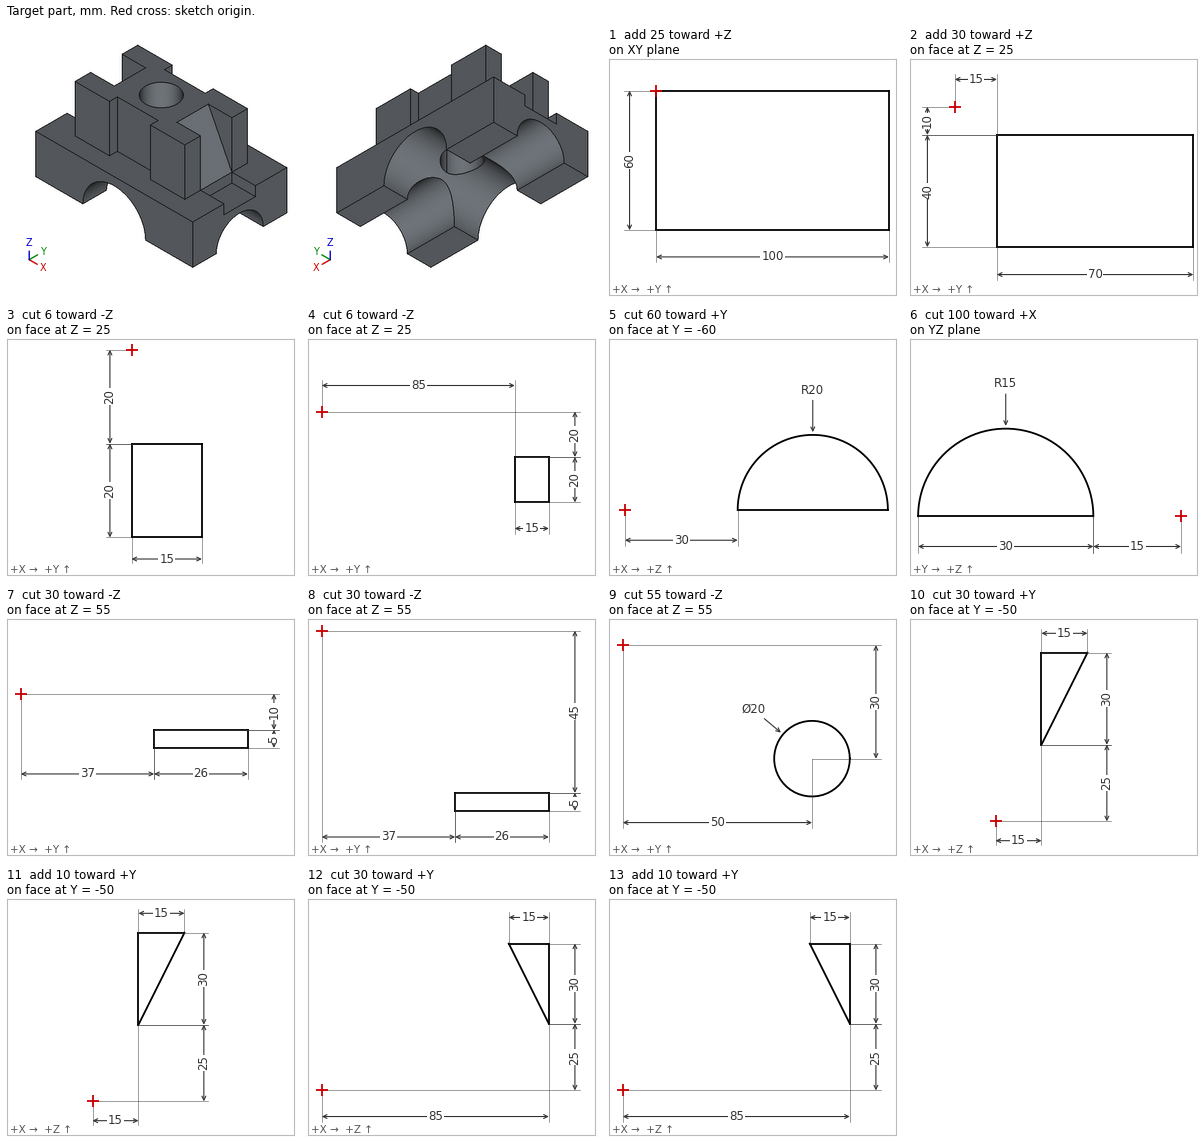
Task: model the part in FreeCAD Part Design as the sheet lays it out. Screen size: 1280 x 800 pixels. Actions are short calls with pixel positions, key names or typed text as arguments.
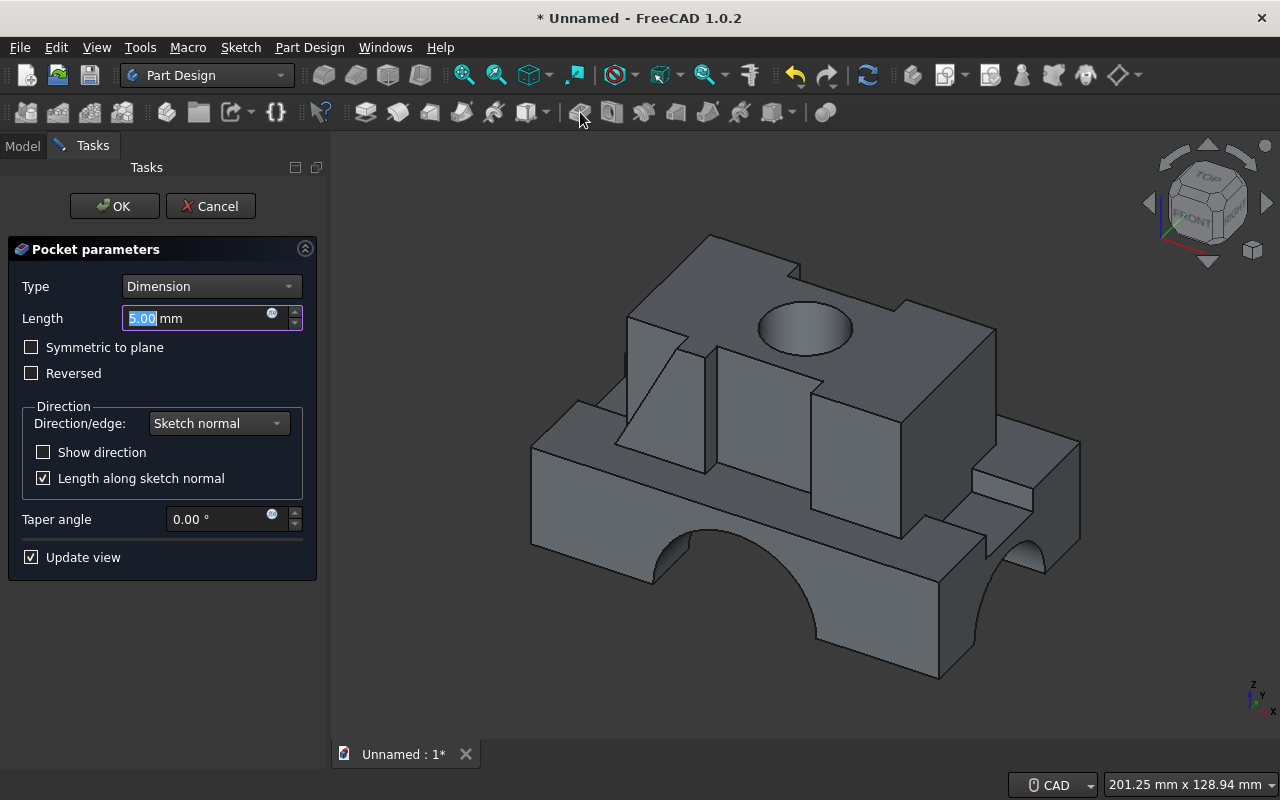
text(30)
key(Tab)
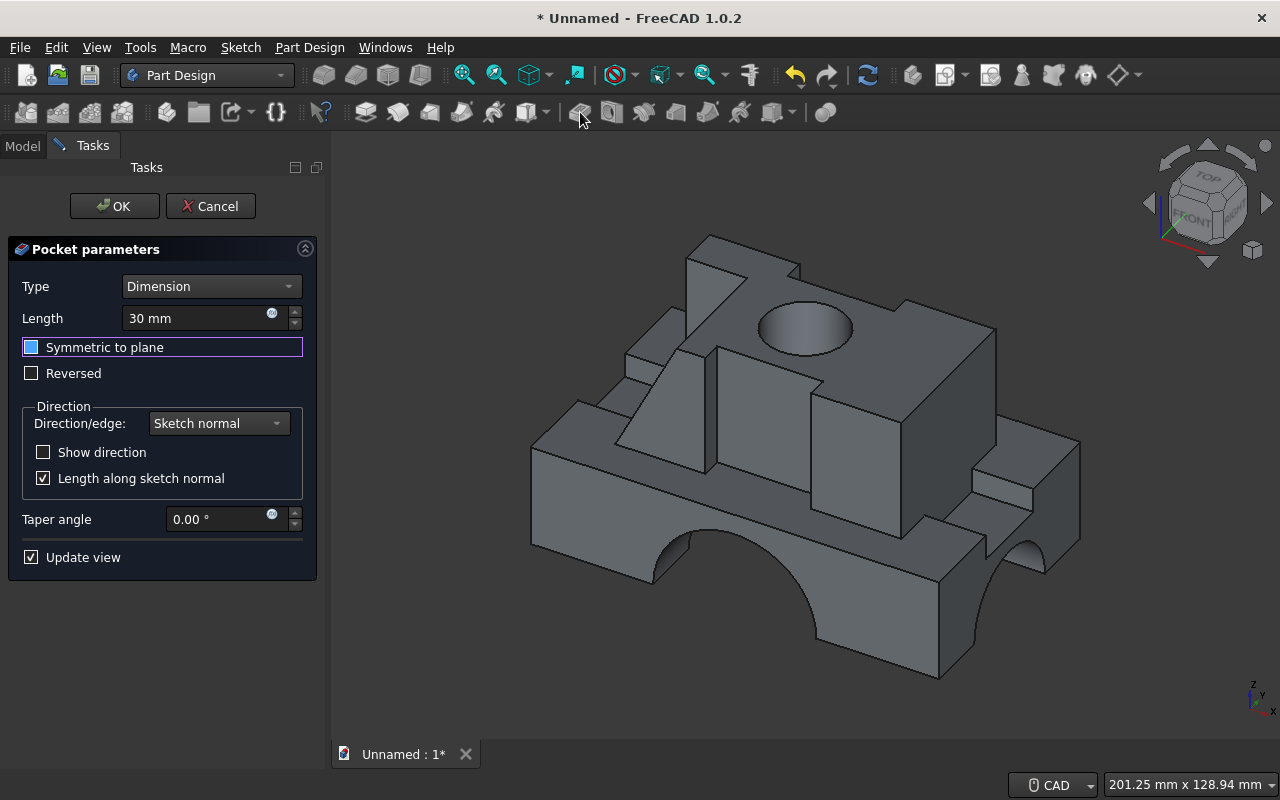
click(115, 206)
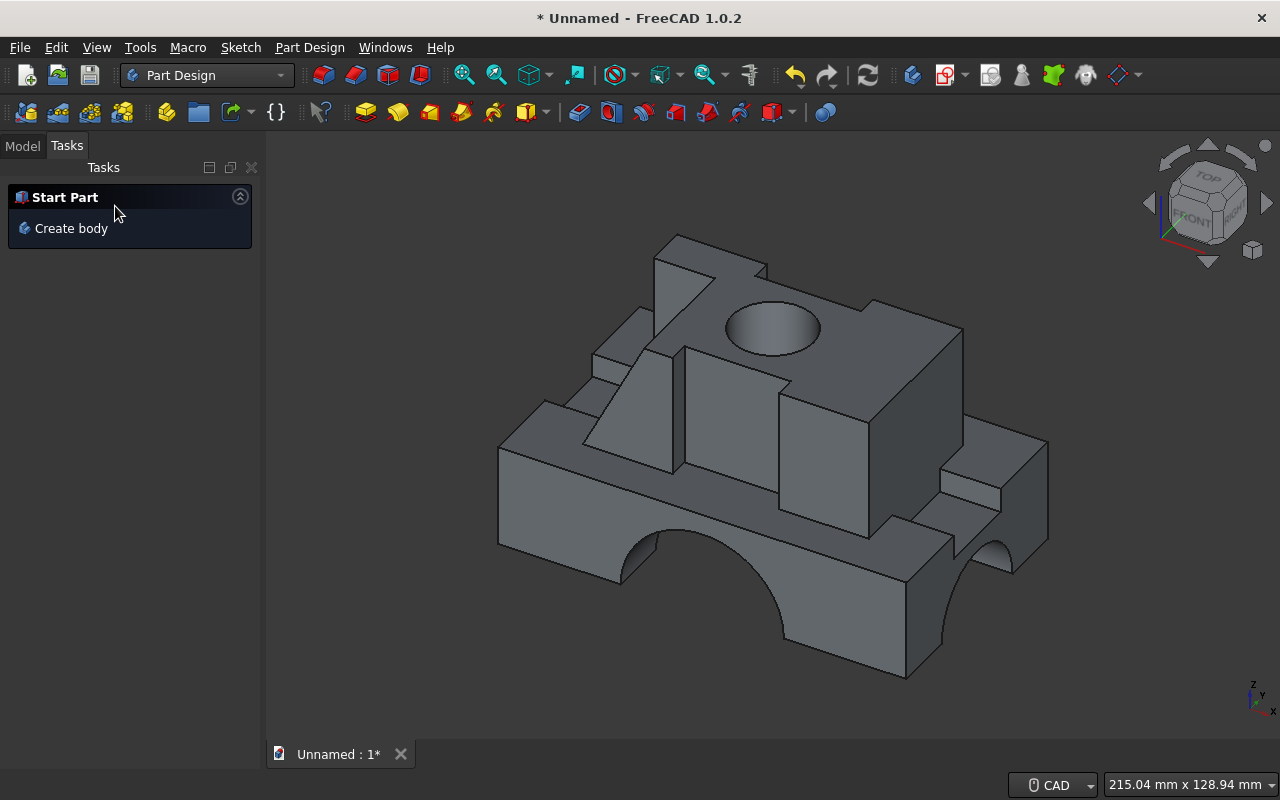
click(824, 465)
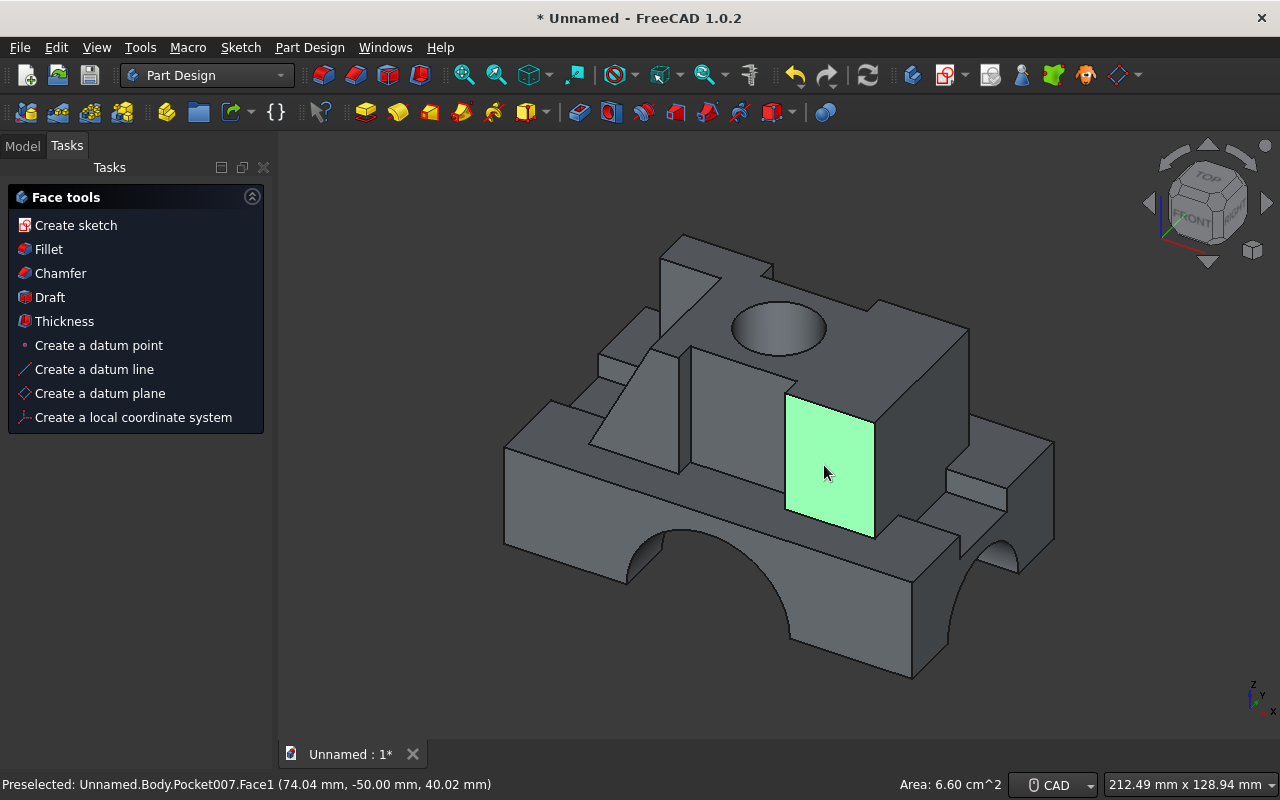
click(946, 76)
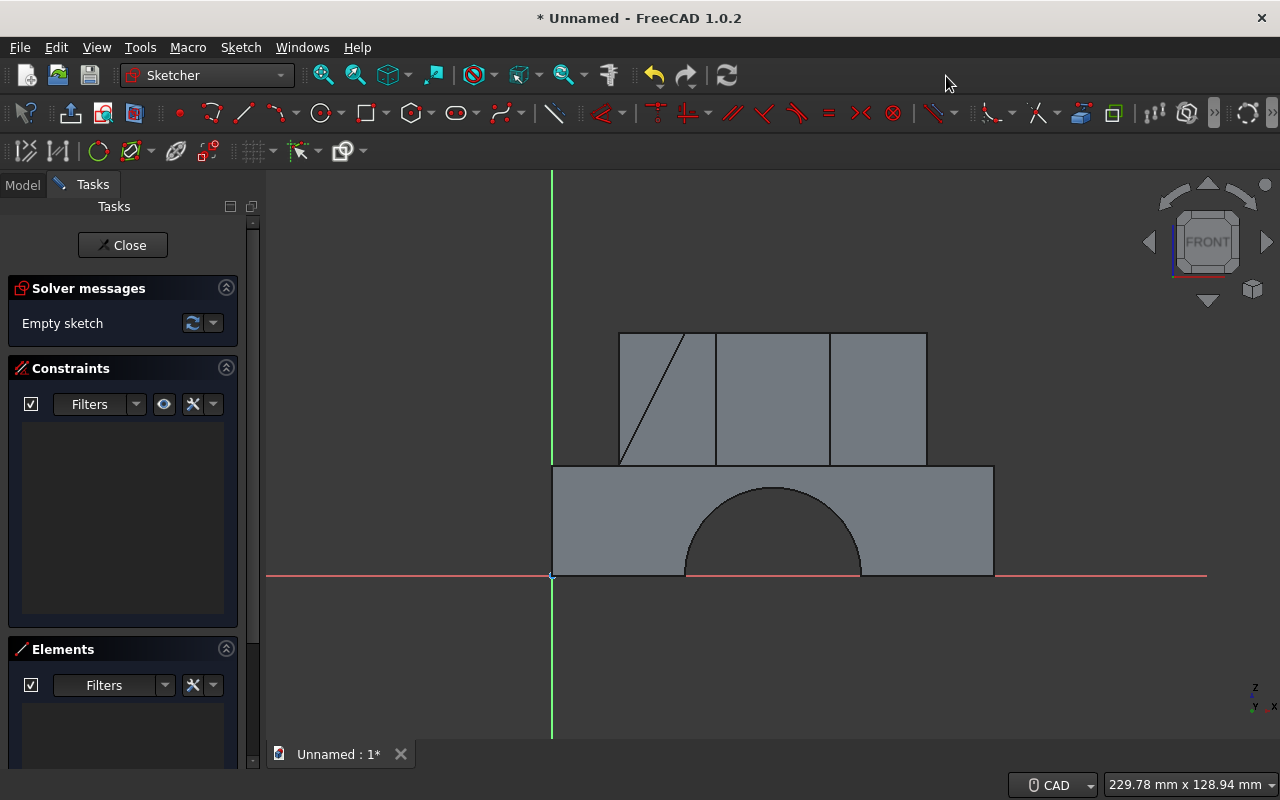
key(q)
key(s)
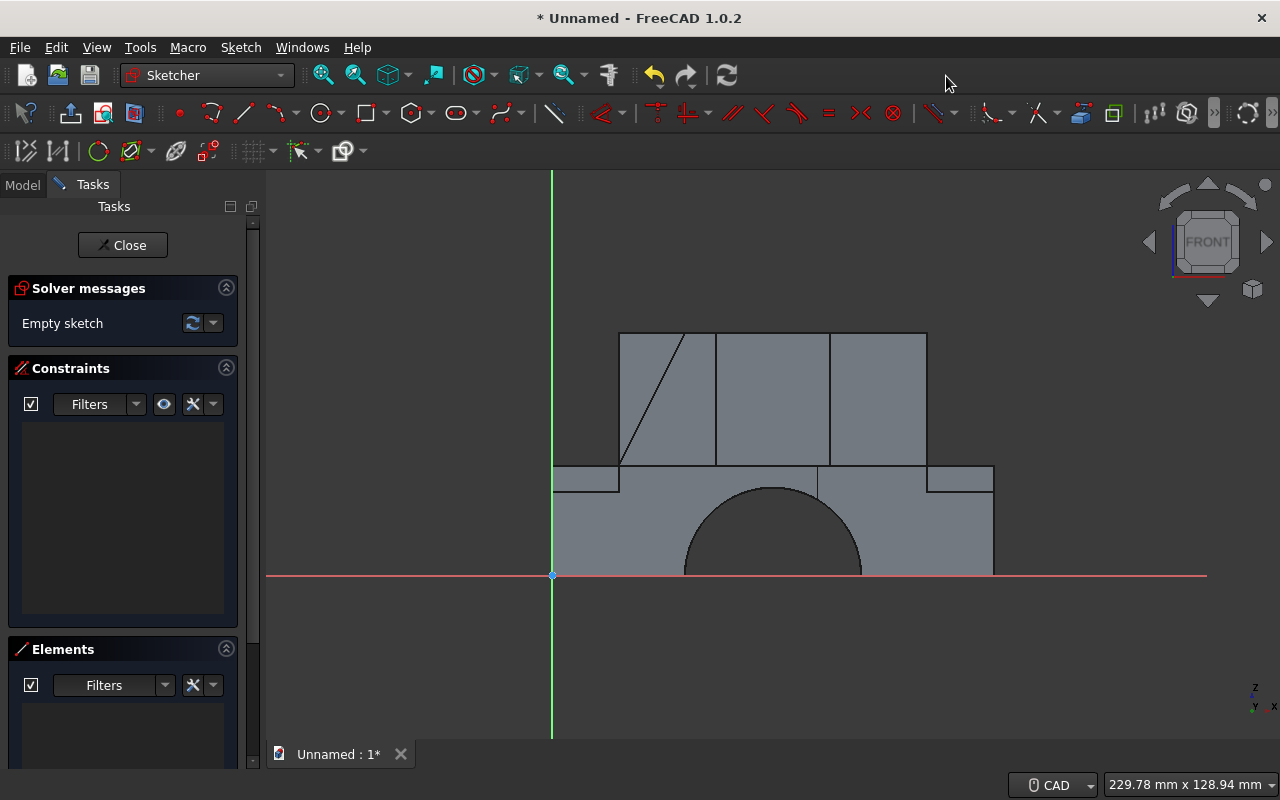
scroll(444, 454, up, 2)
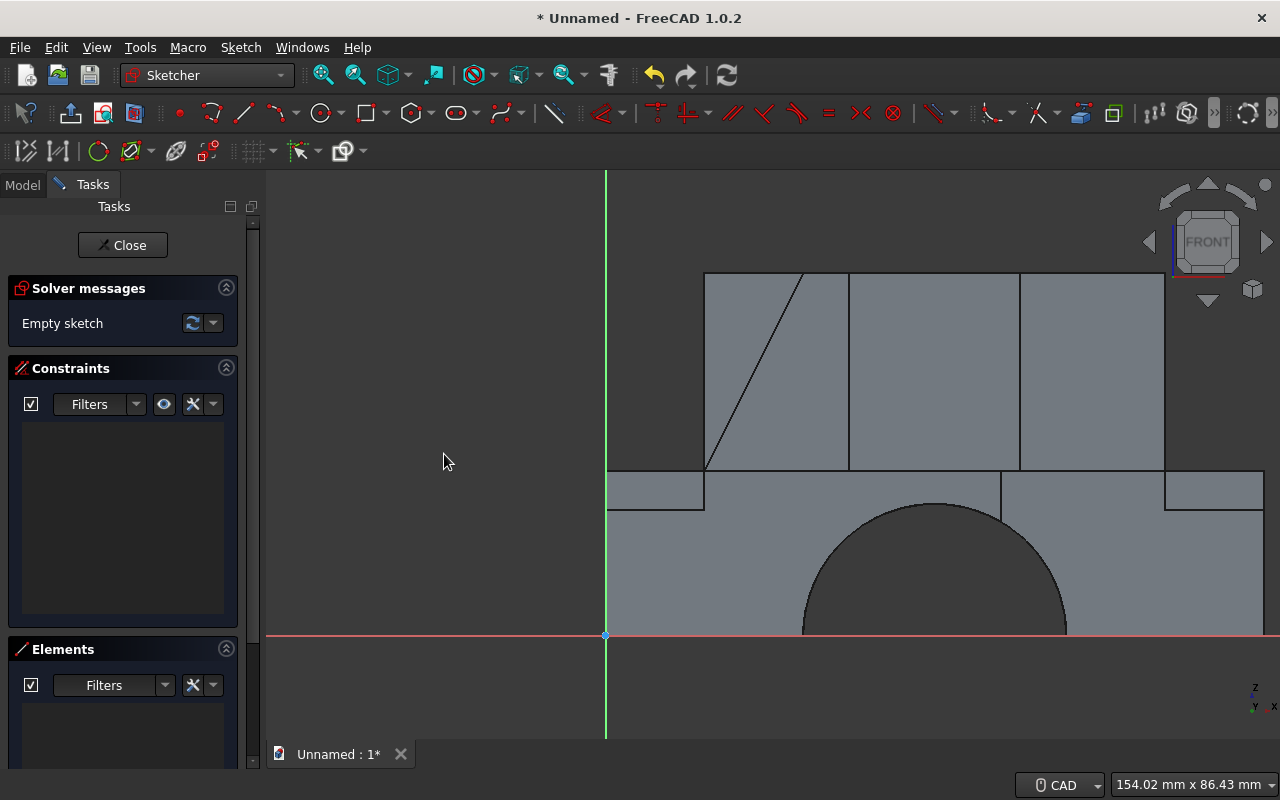
key(g)
key(m)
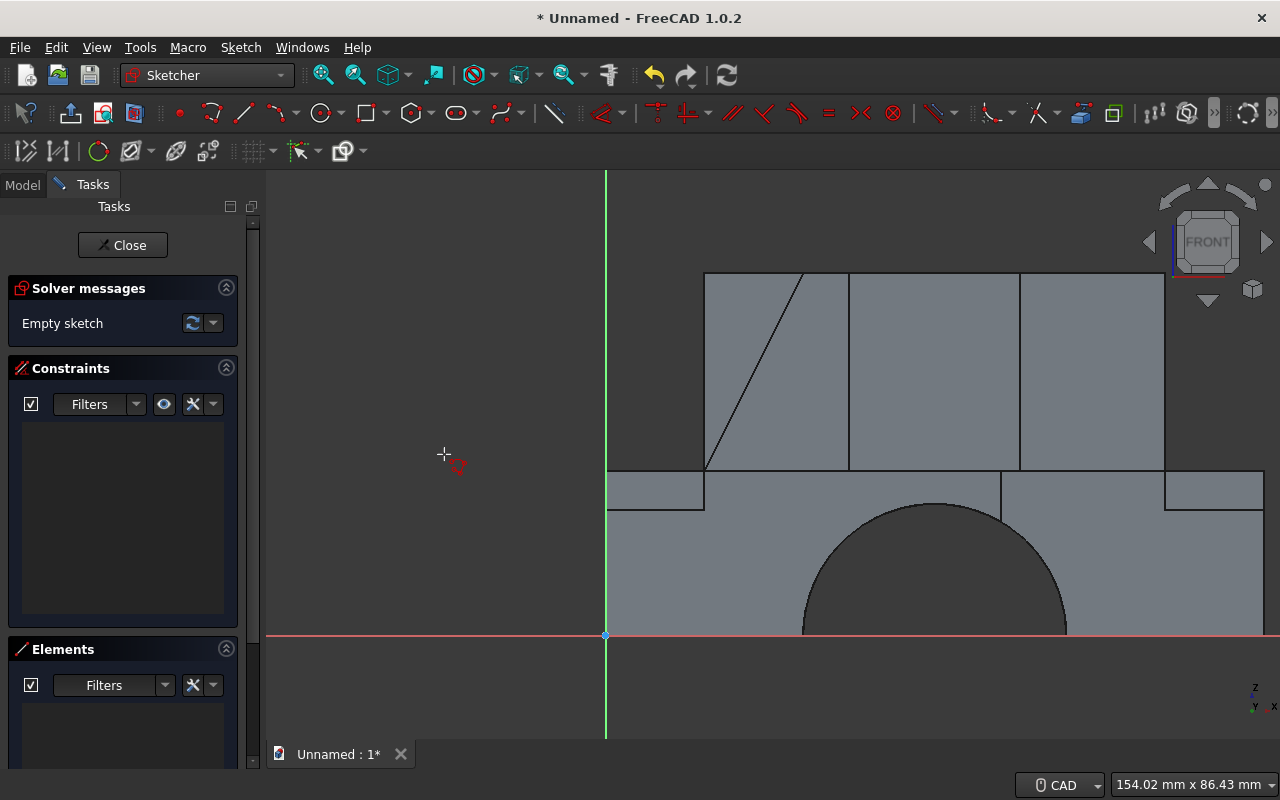
click(704, 471)
click(803, 273)
click(704, 273)
click(704, 472)
key(Escape)
key(Escape)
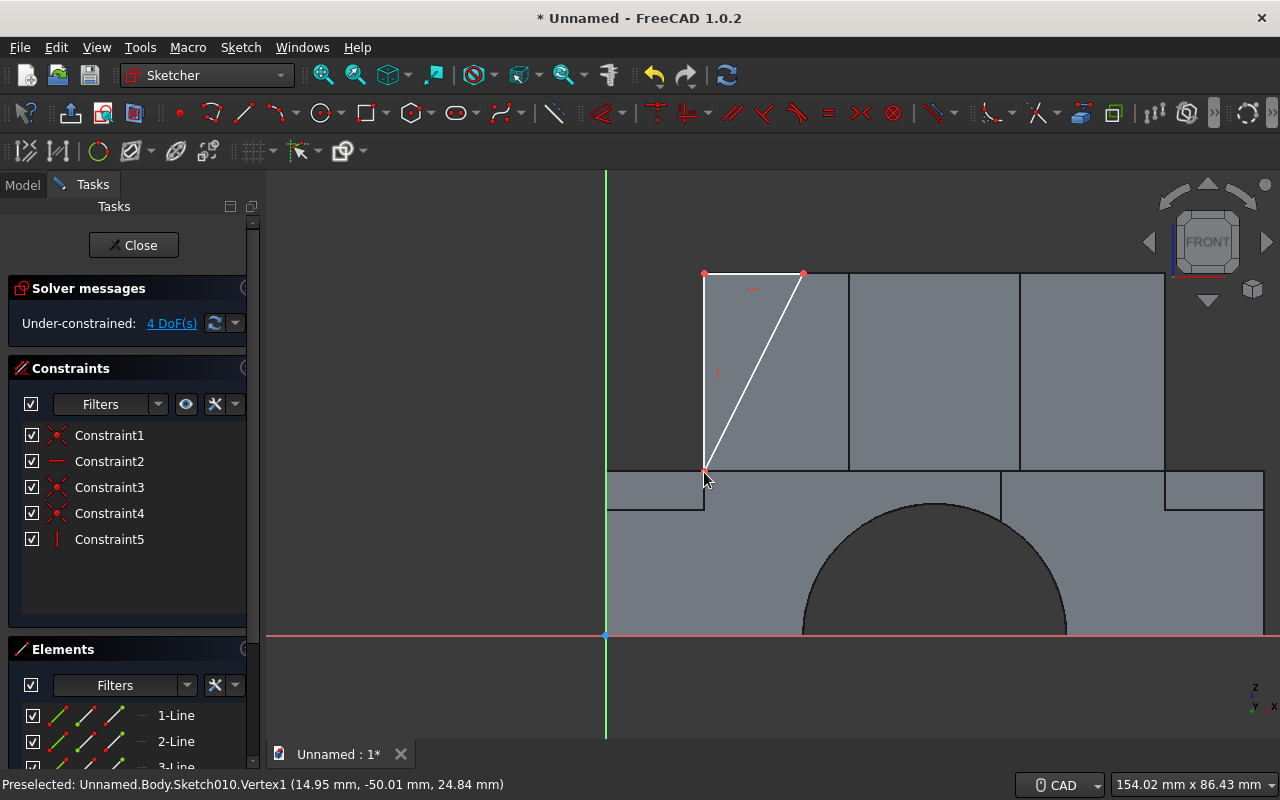
key(d)